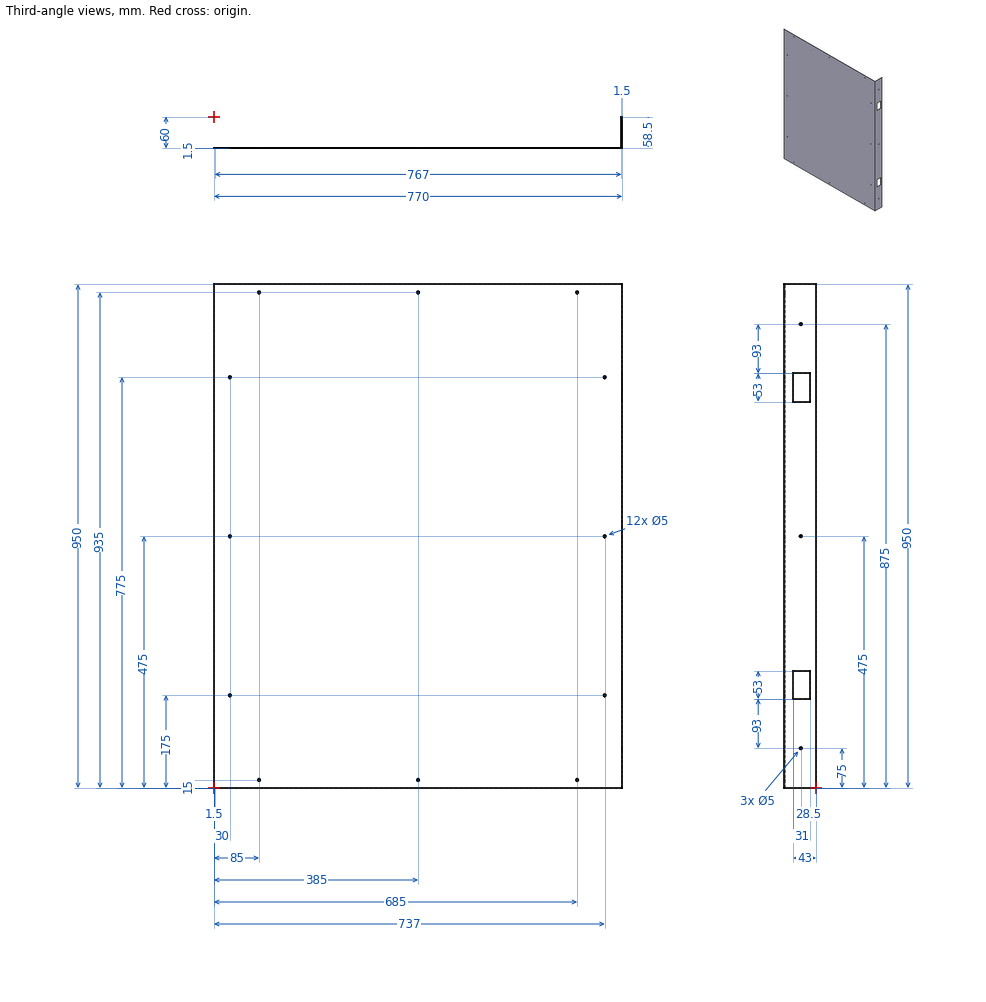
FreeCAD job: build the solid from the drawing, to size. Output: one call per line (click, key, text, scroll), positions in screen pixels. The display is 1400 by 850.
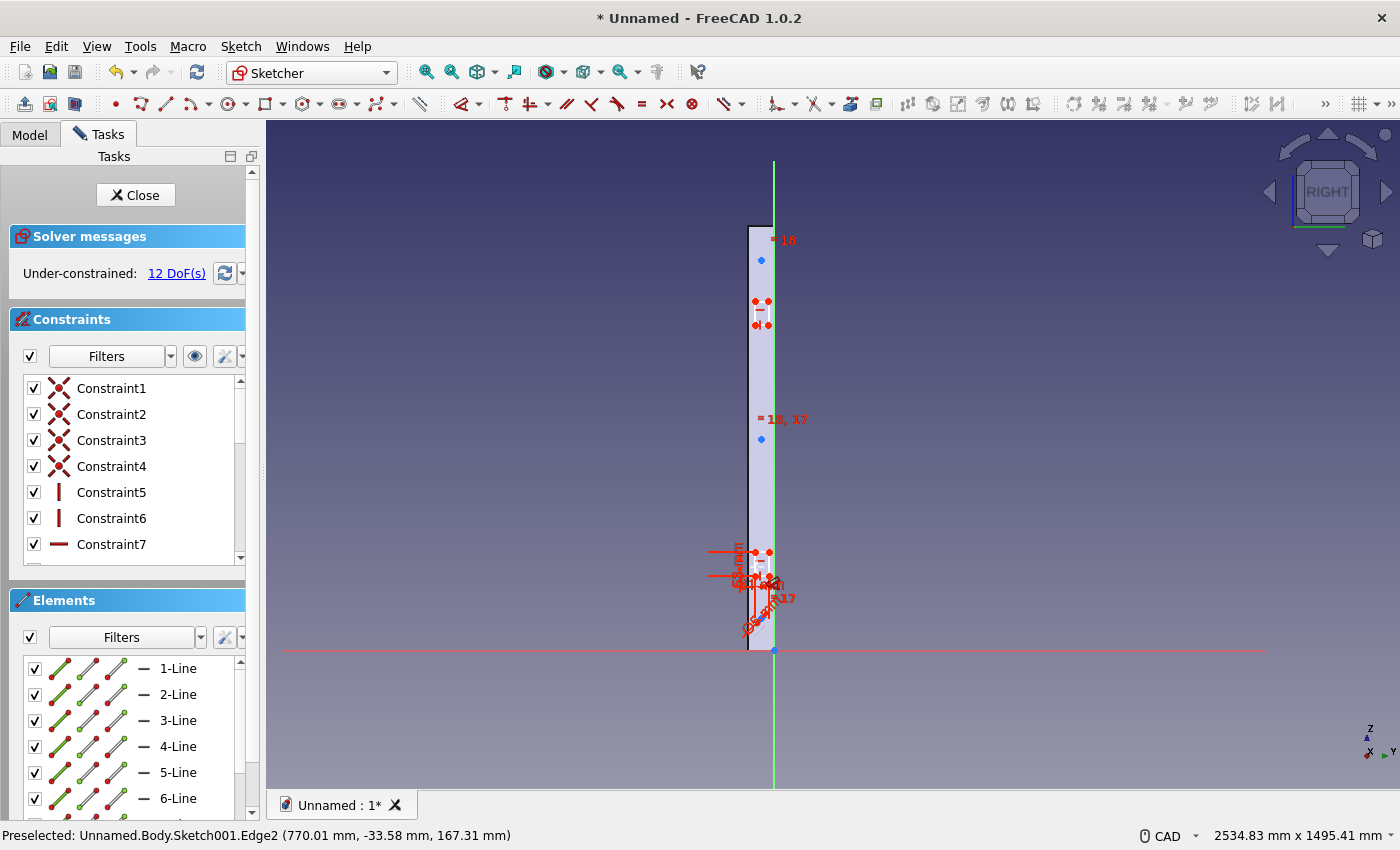
scroll(755, 309, up, 4)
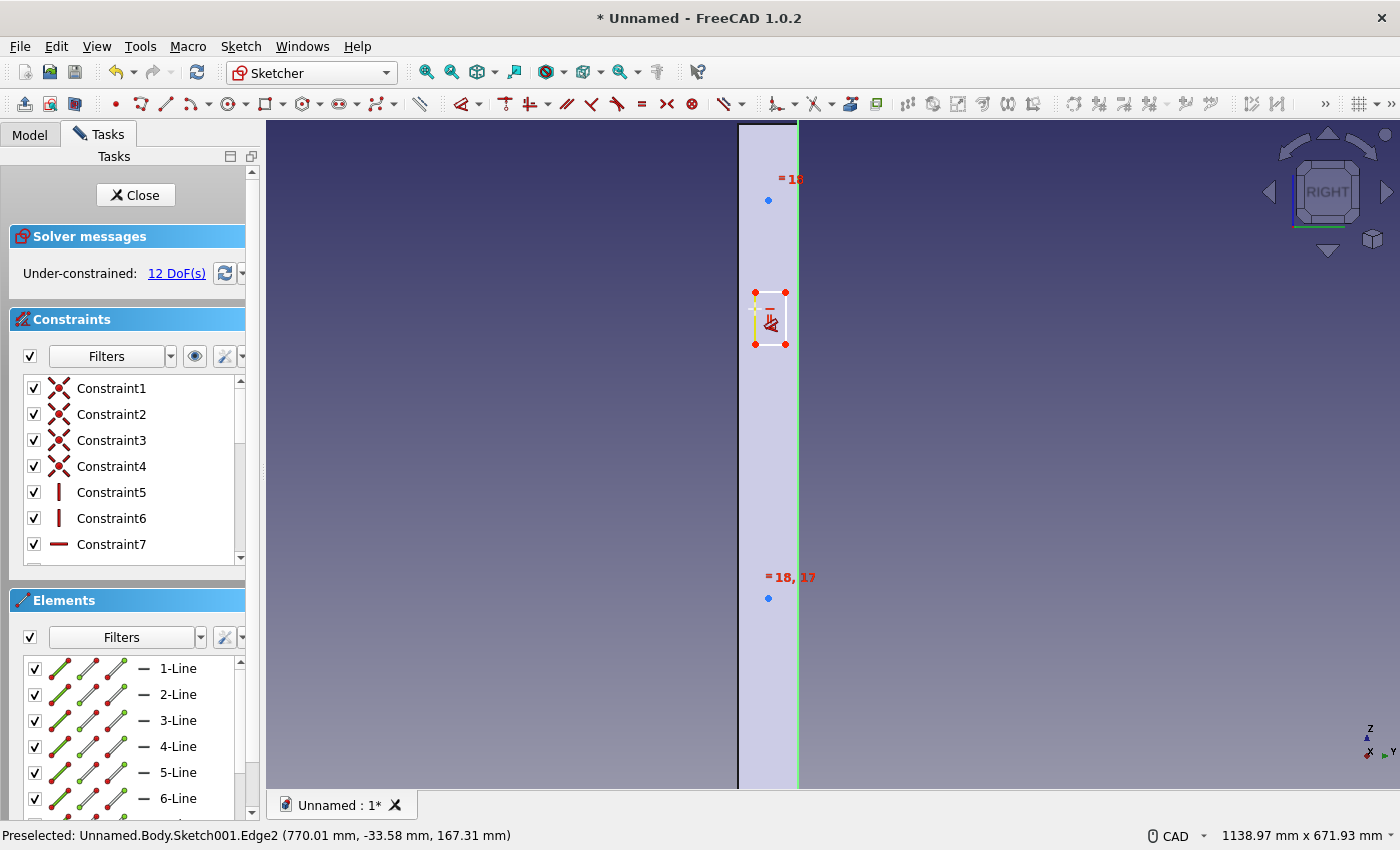
click(755, 308)
click(721, 318)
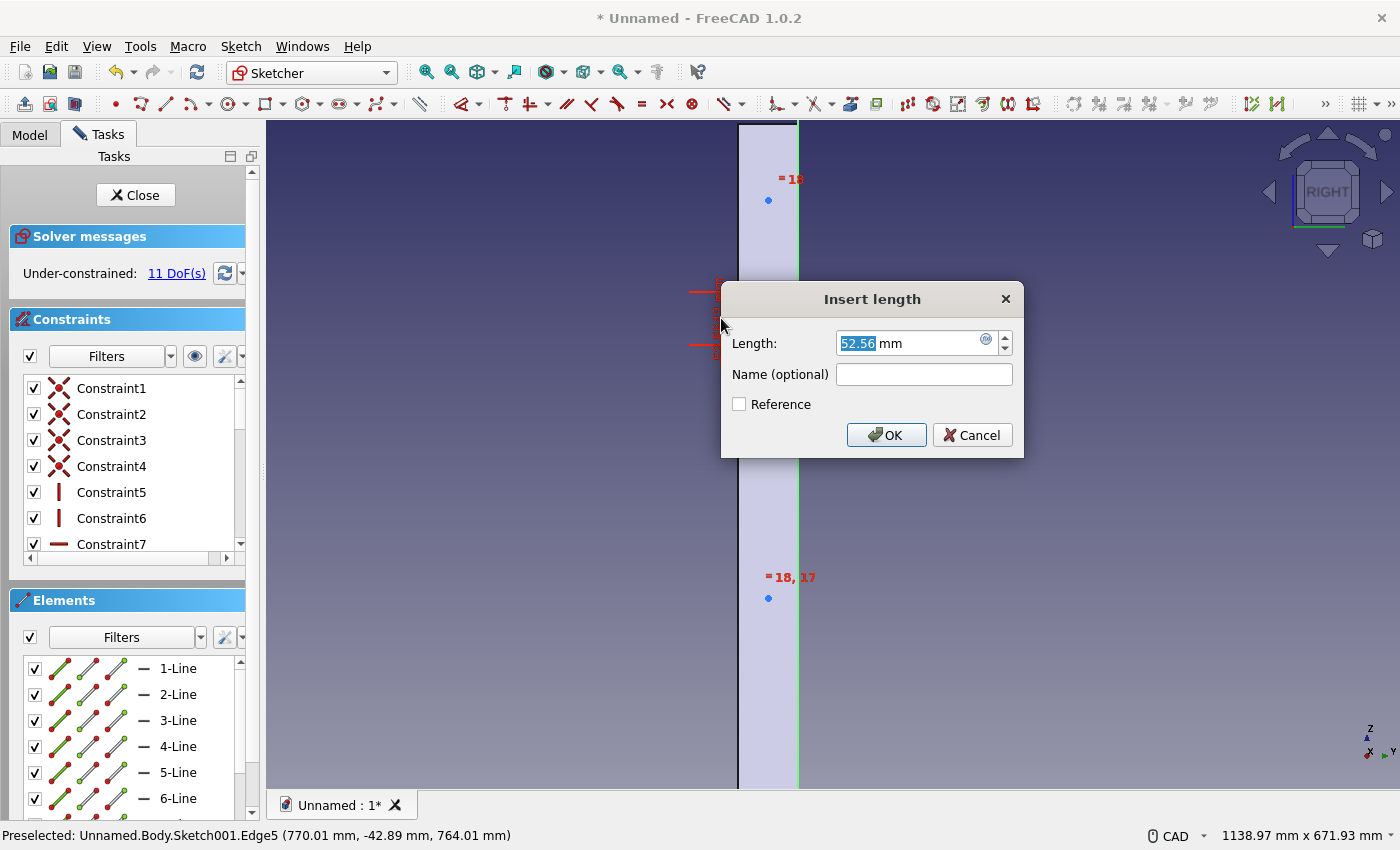
text(53)
key(Return)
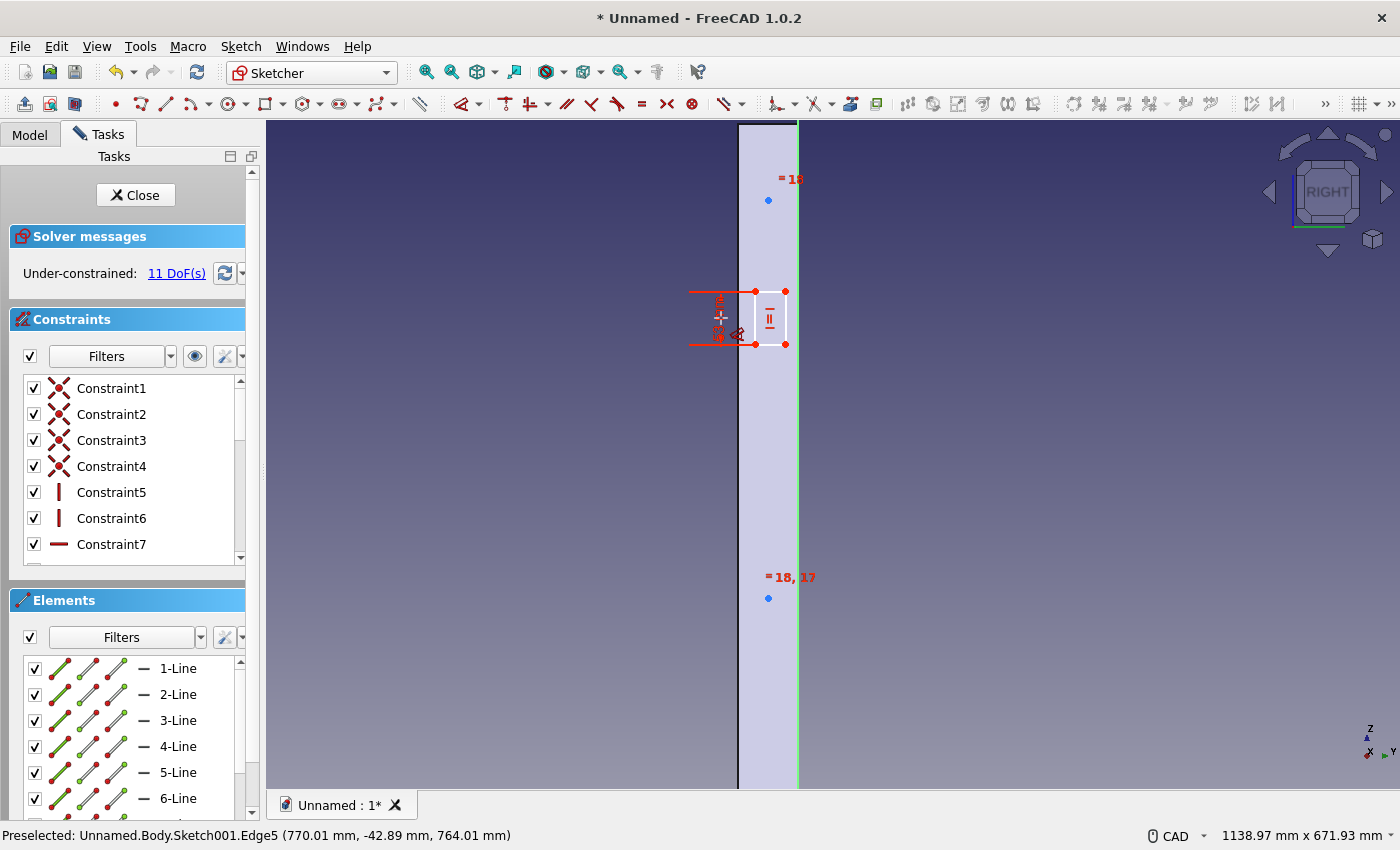
scroll(764, 345, up, 3)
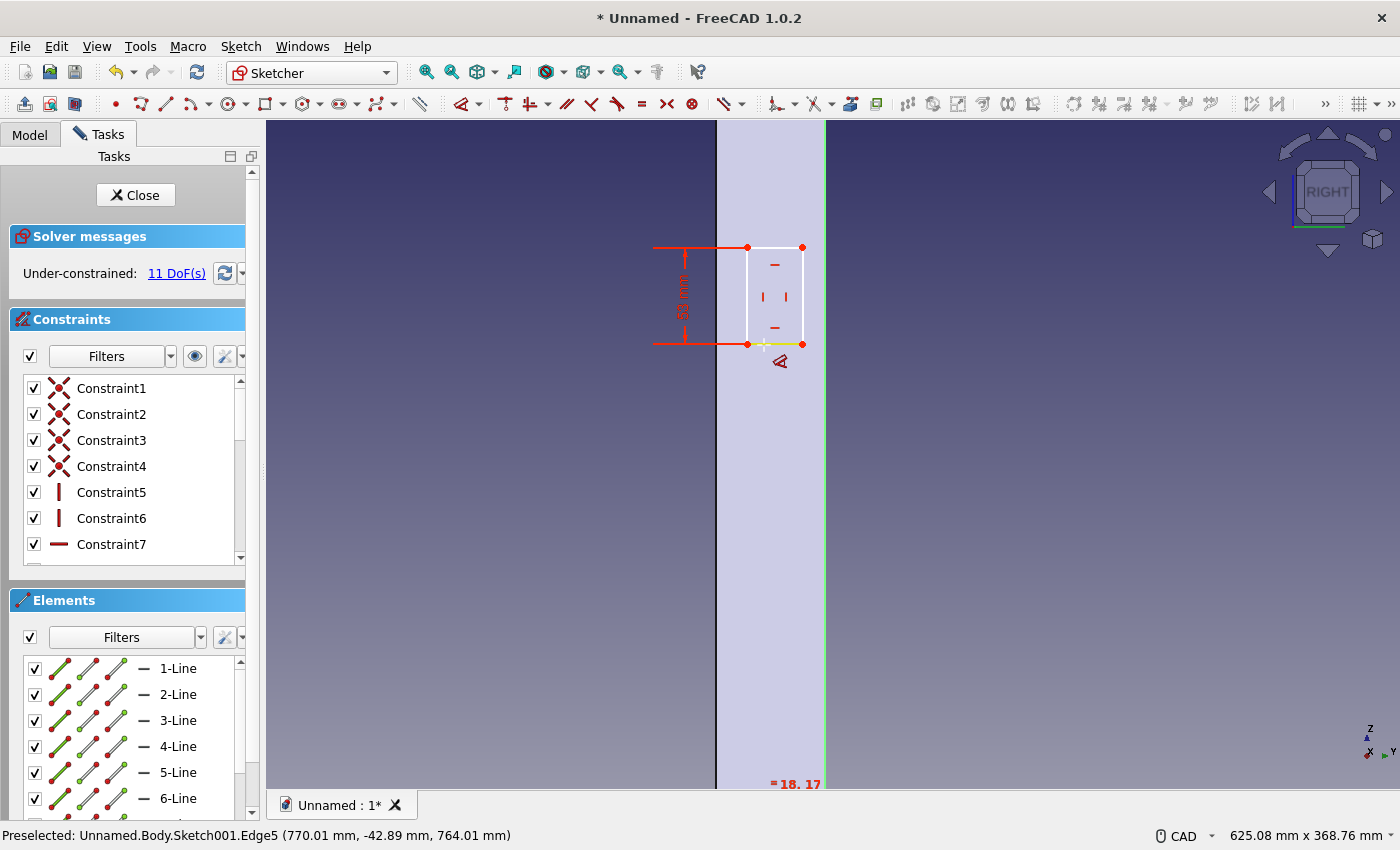
click(764, 344)
click(775, 310)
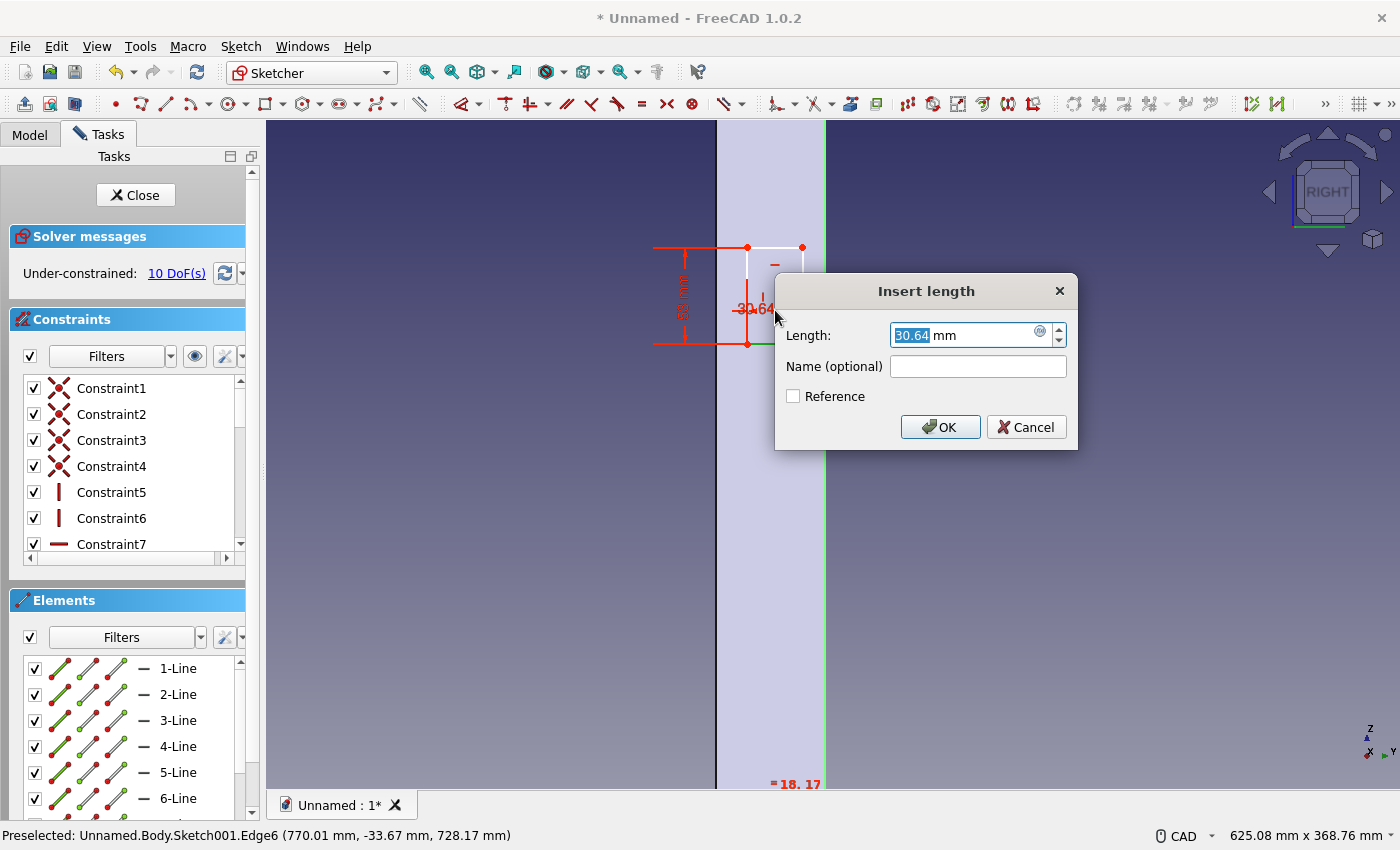
text(31)
key(Return)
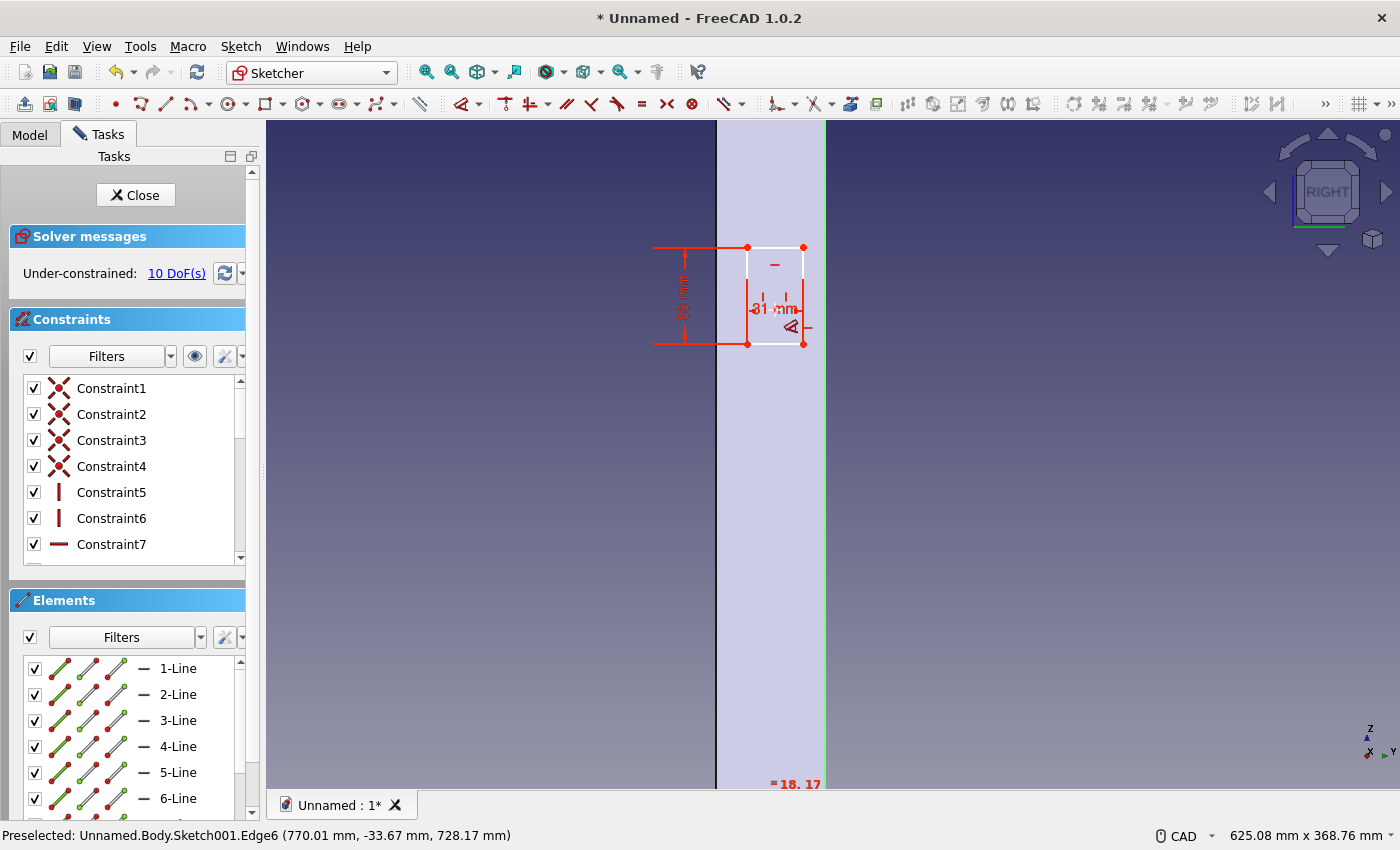
scroll(757, 319, down, 7)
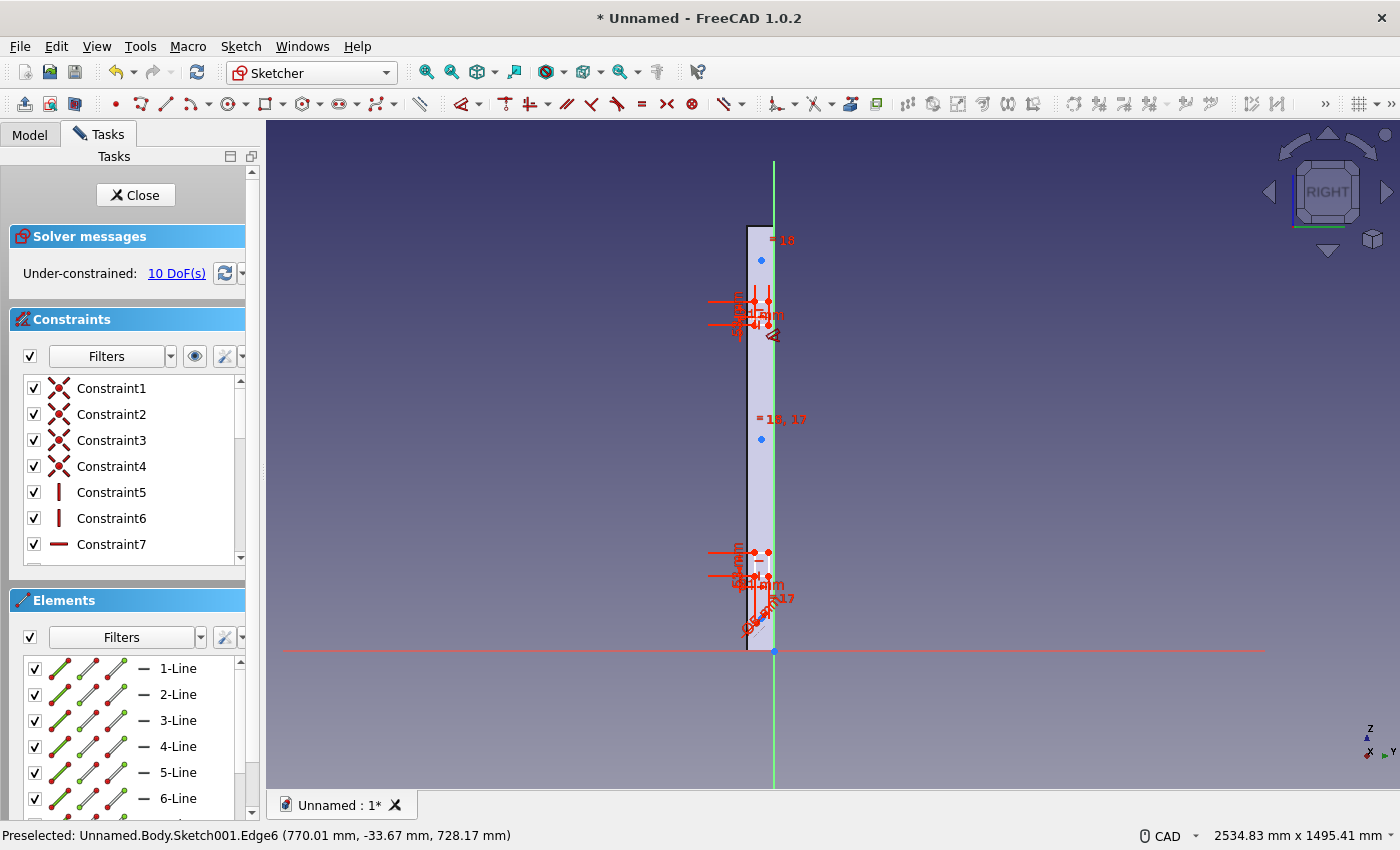
click(761, 619)
click(856, 635)